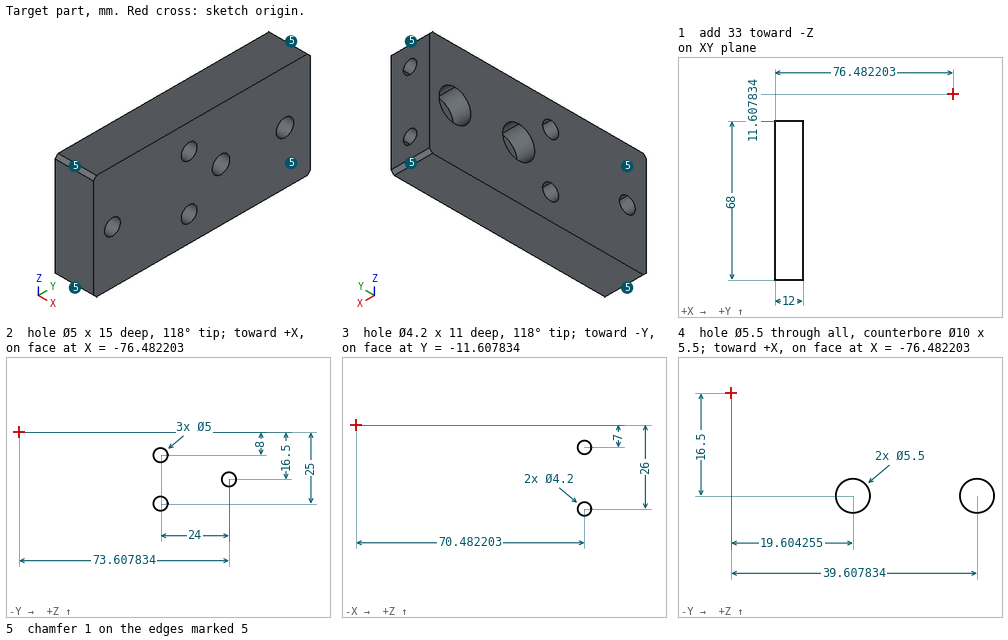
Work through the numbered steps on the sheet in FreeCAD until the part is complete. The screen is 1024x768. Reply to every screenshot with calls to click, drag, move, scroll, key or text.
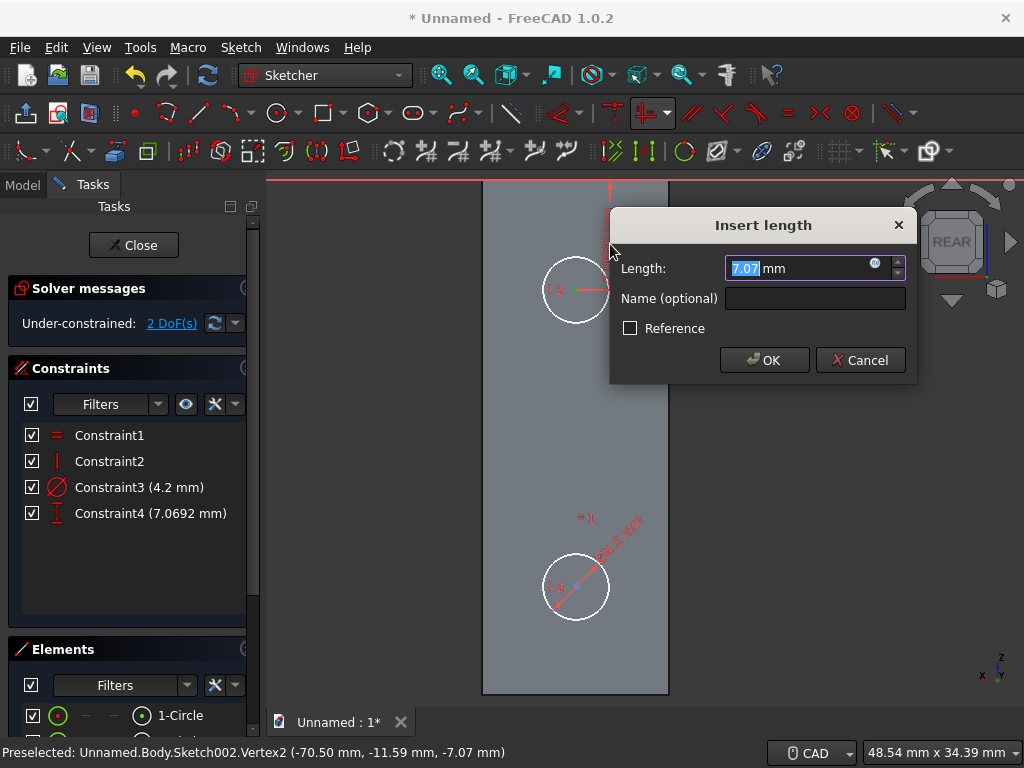
text(7)
key(Return)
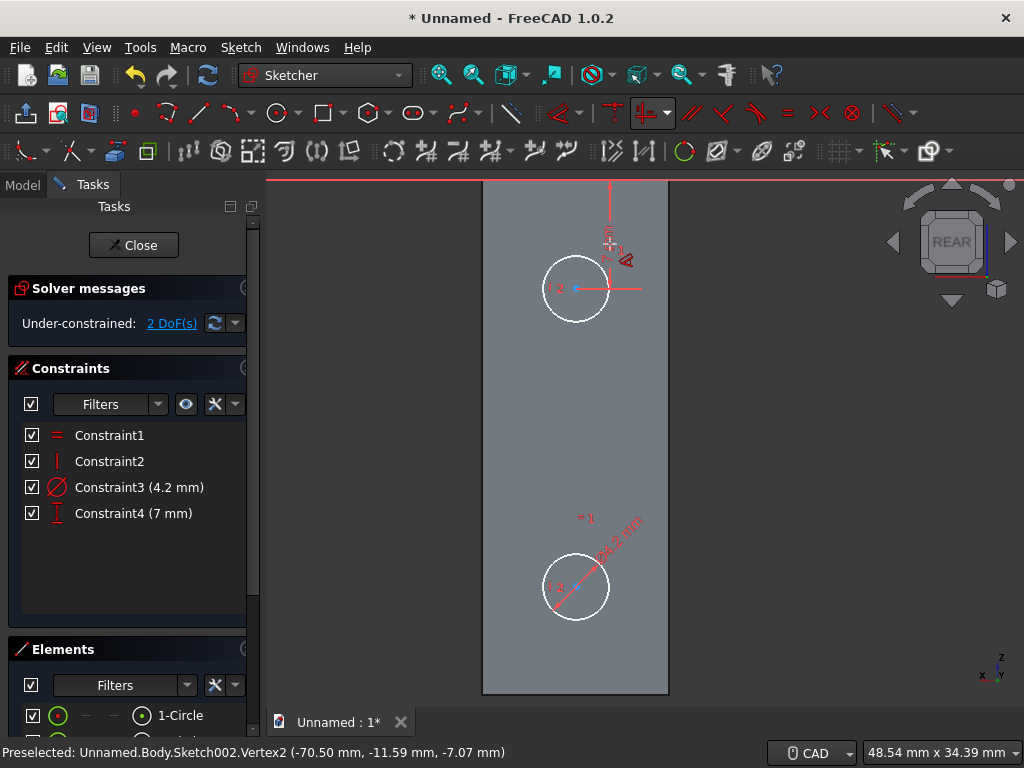
click(576, 587)
click(610, 392)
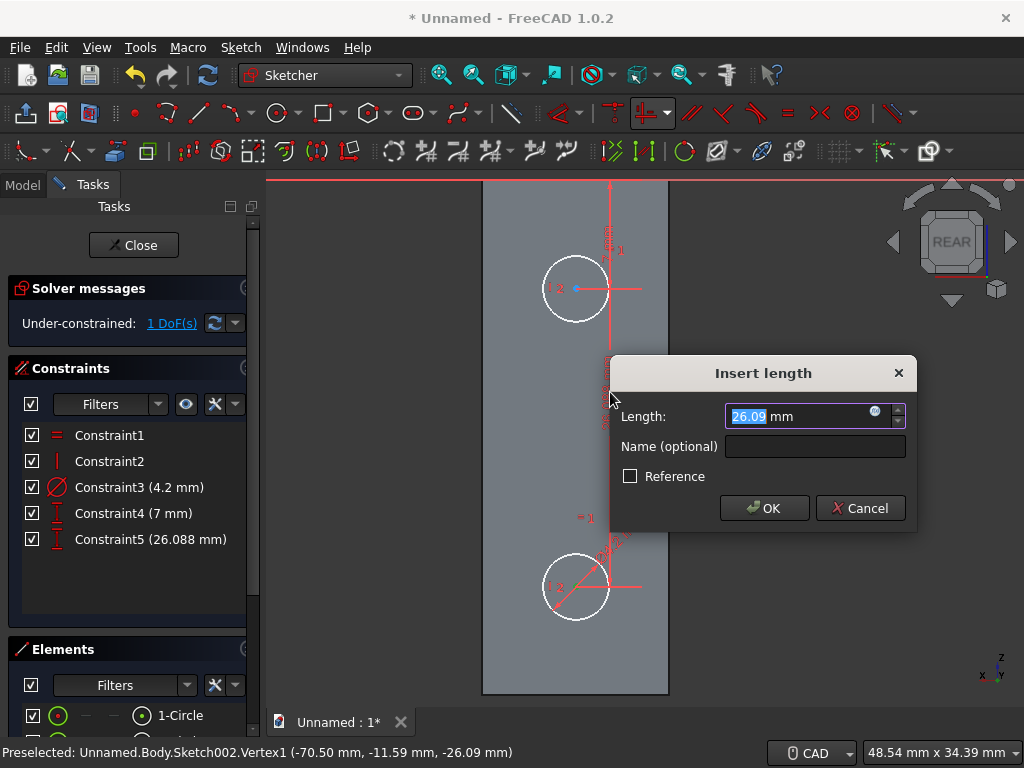
text(26)
key(Return)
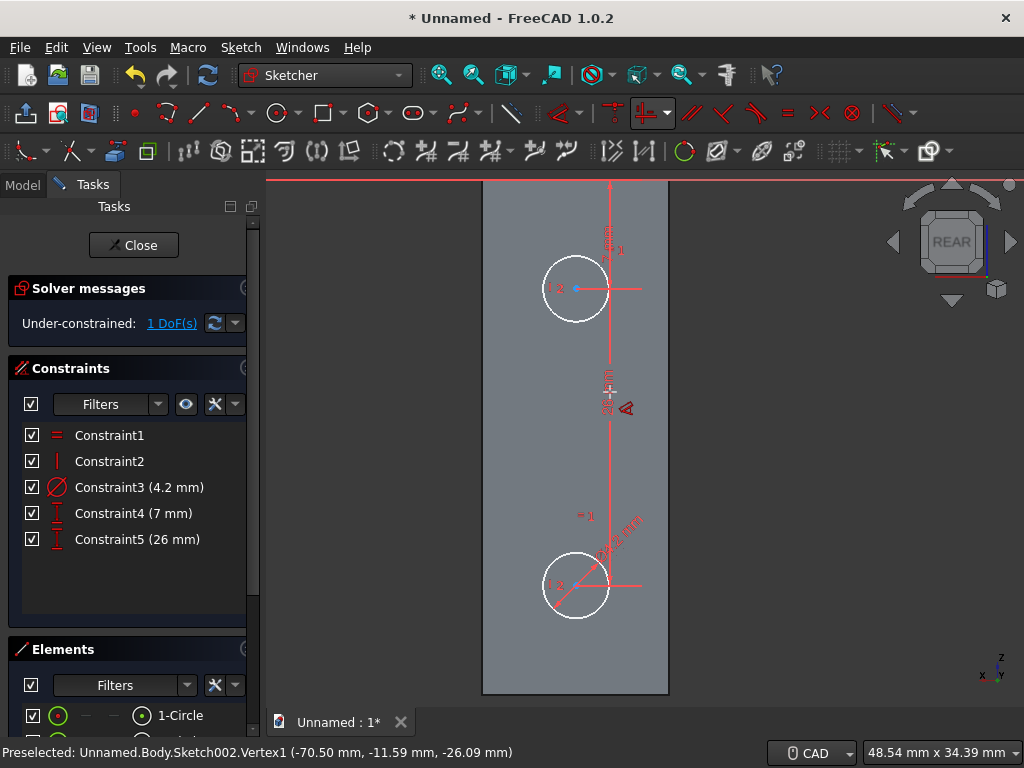
click(576, 586)
click(435, 620)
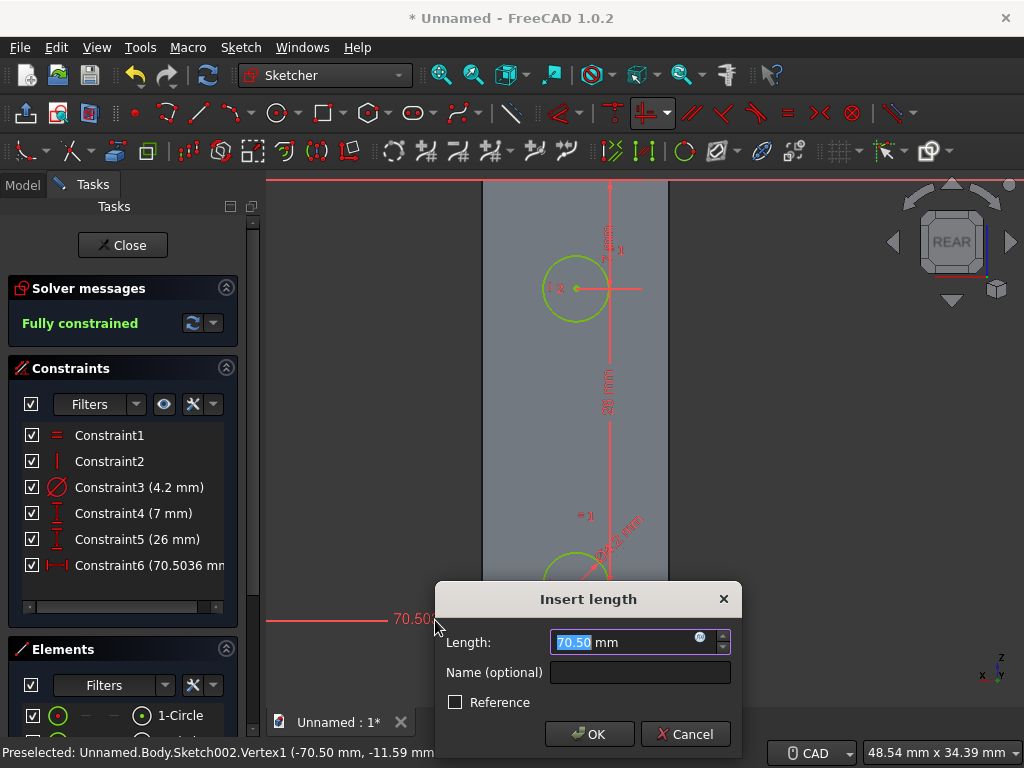
text(70.482203)
key(Return)
key(Escape)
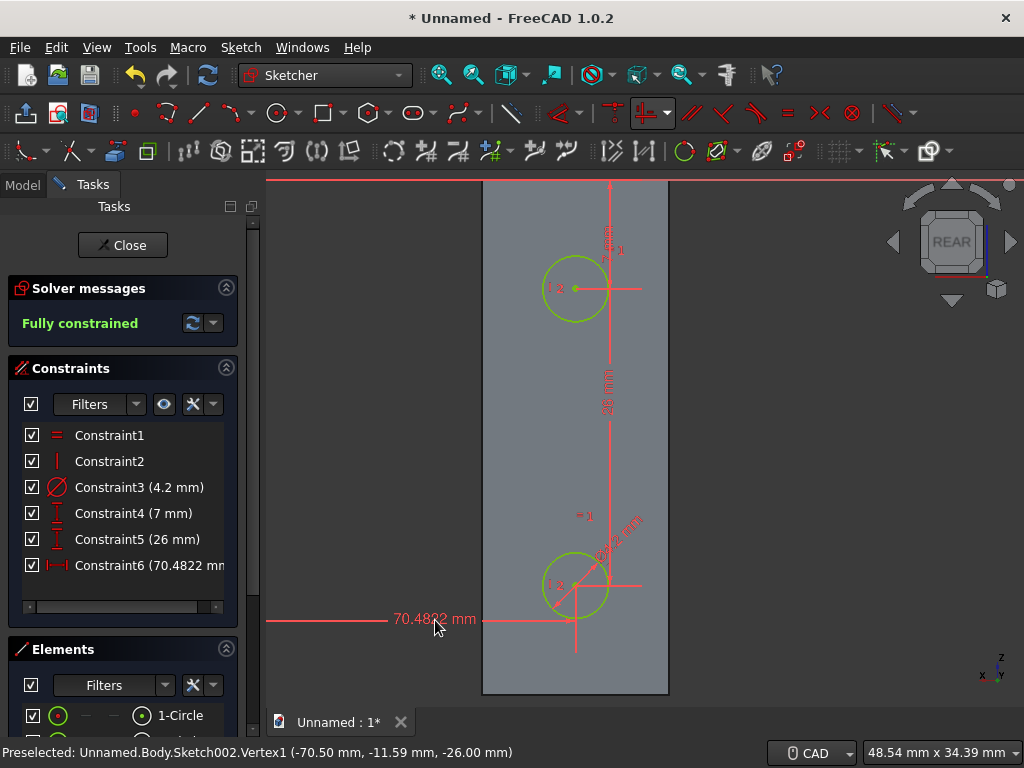
click(123, 245)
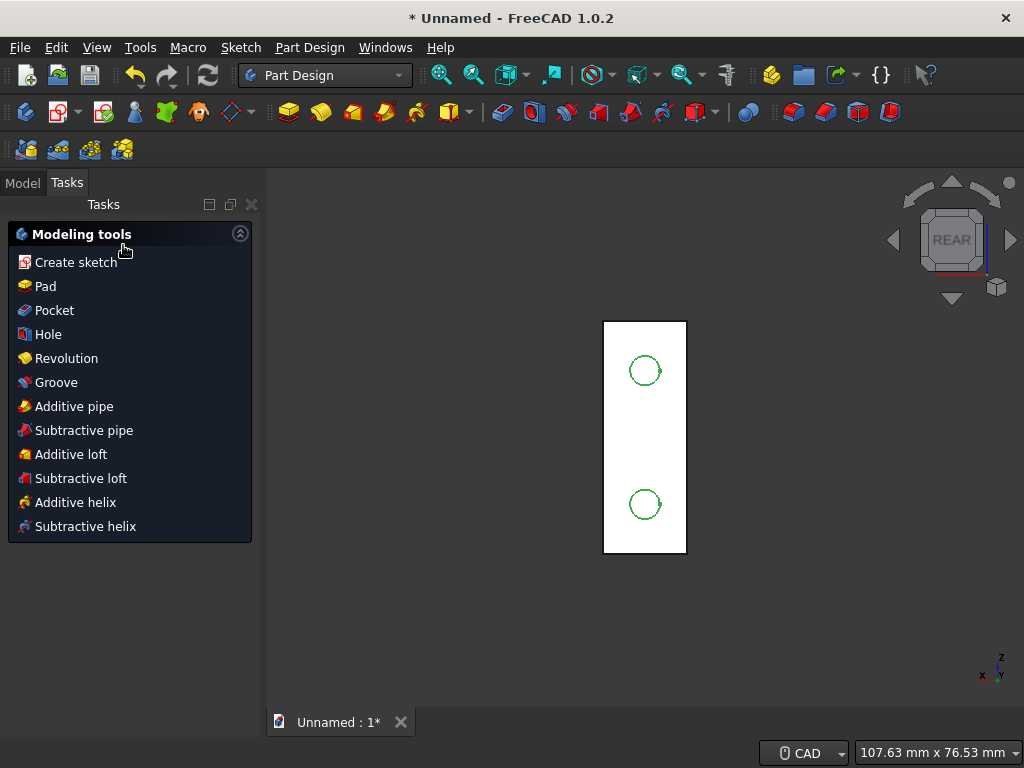
click(536, 112)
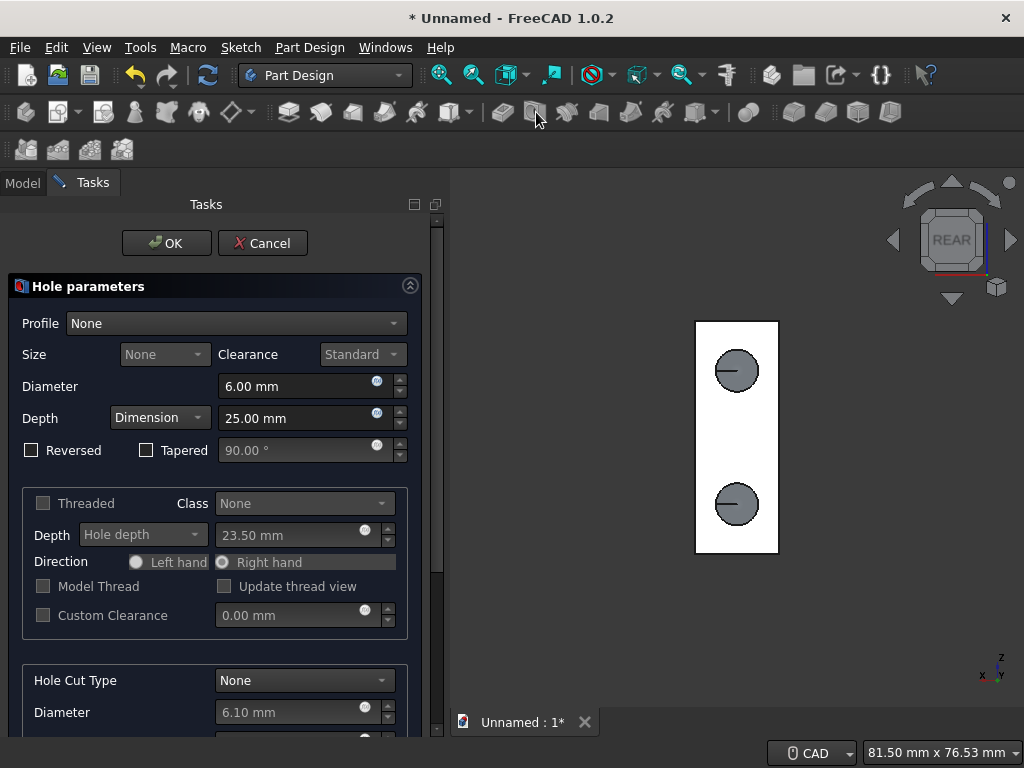
triple_click(305, 386)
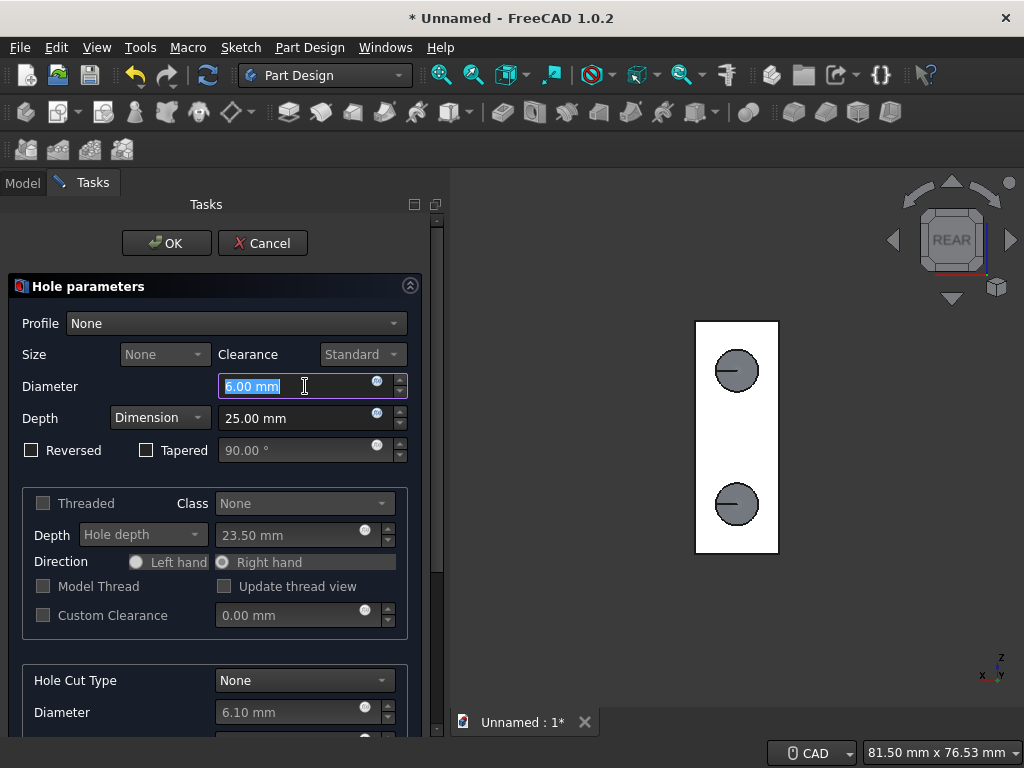
text(4.2)
key(Tab)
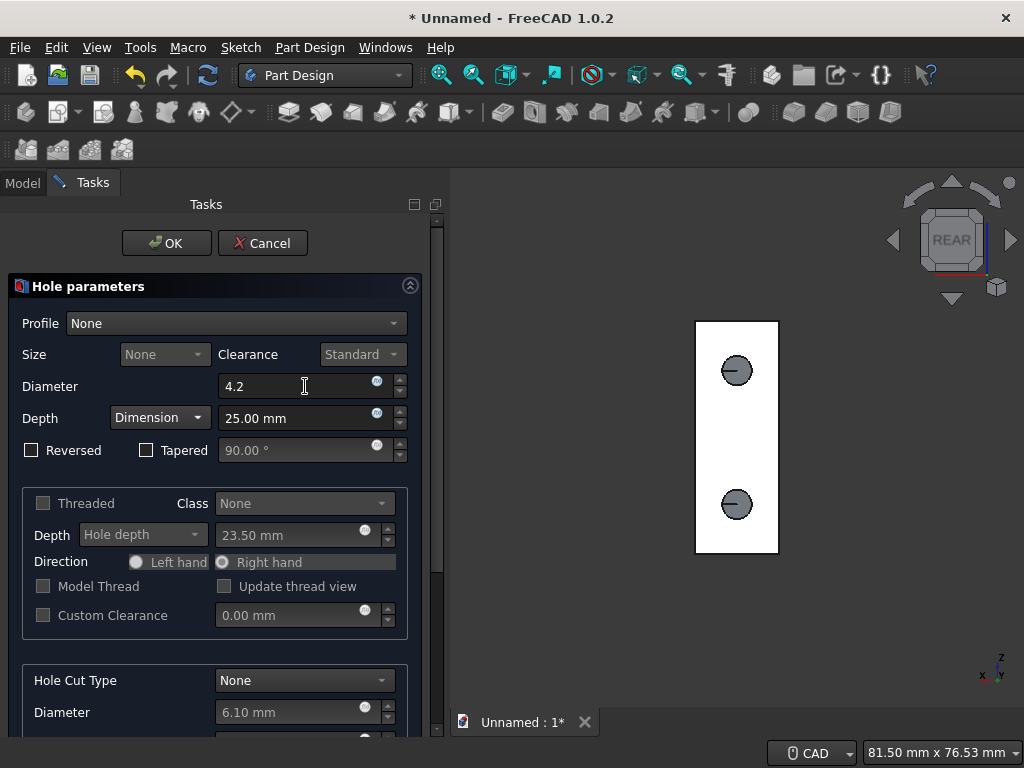
triple_click(305, 418)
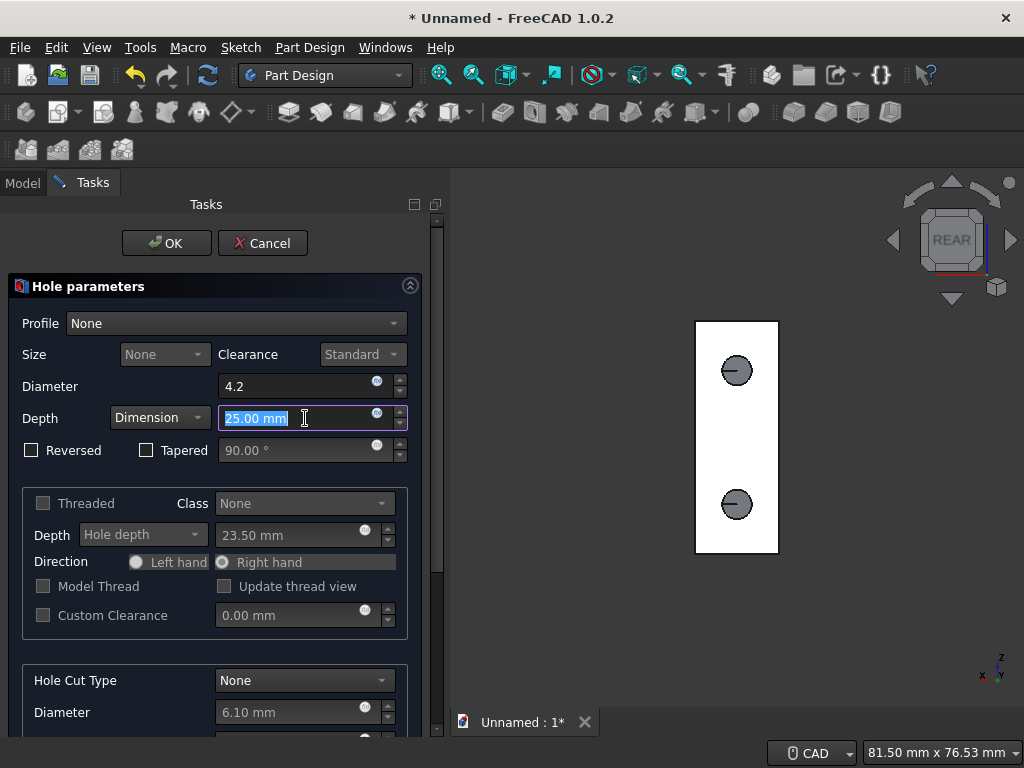
text(11)
key(Tab)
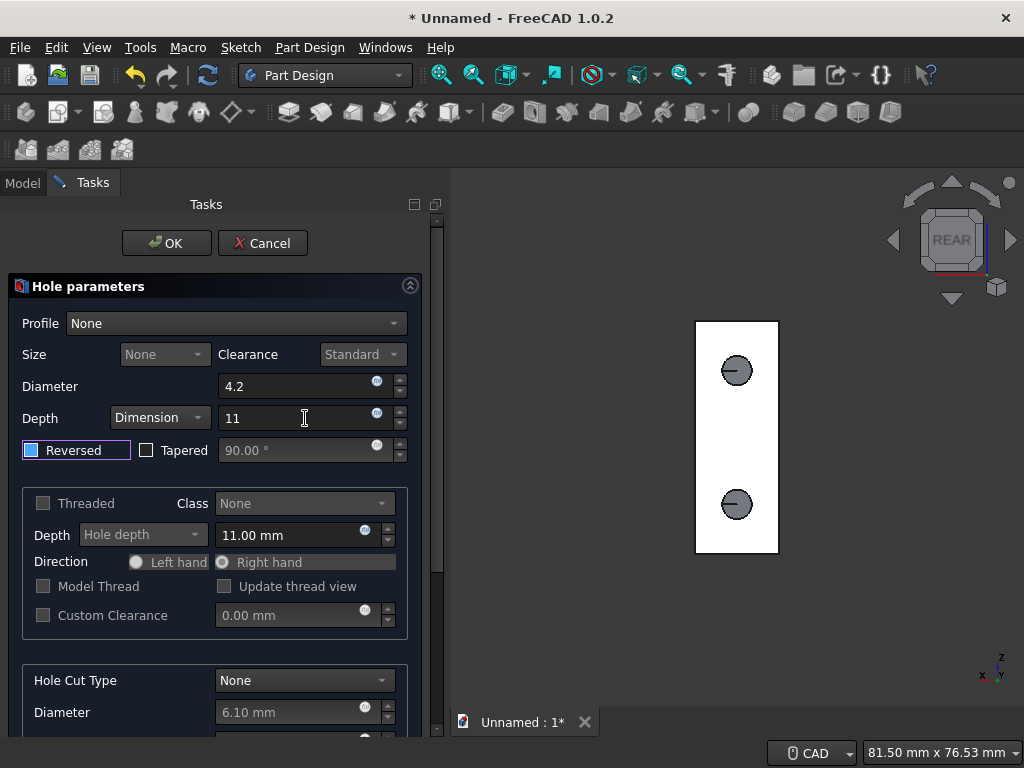
click(167, 243)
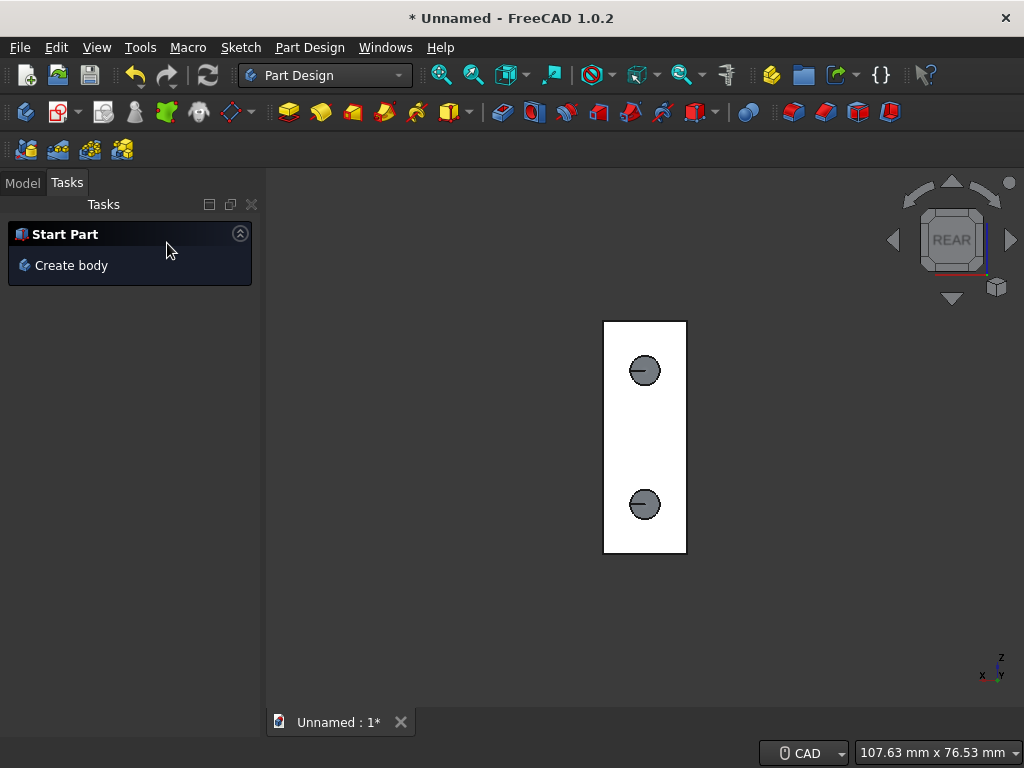
click(442, 76)